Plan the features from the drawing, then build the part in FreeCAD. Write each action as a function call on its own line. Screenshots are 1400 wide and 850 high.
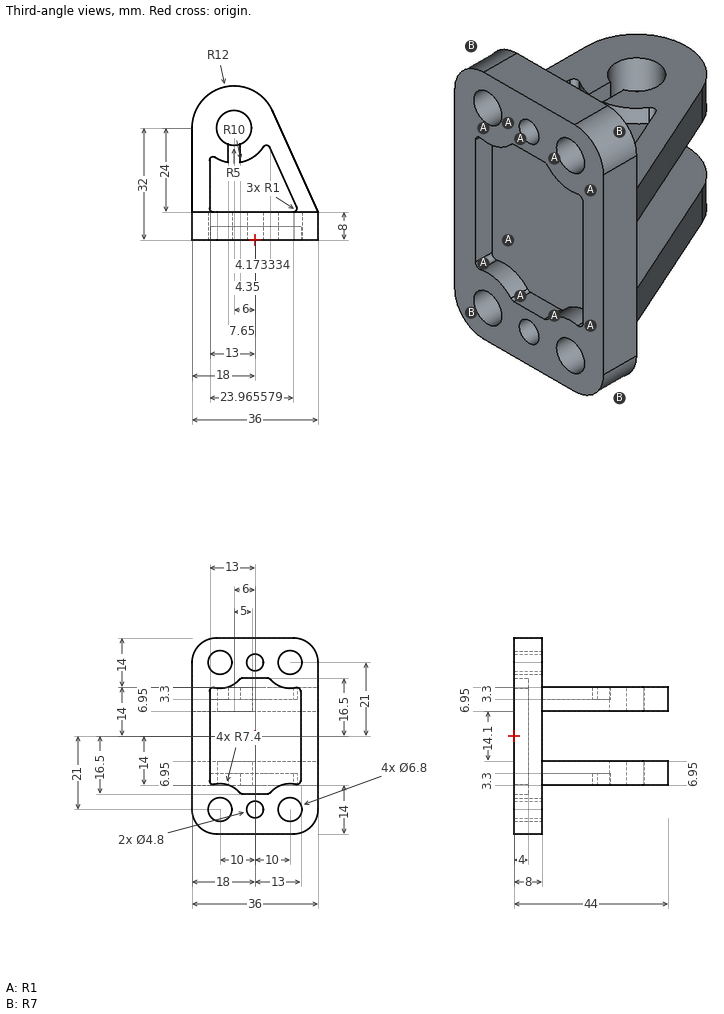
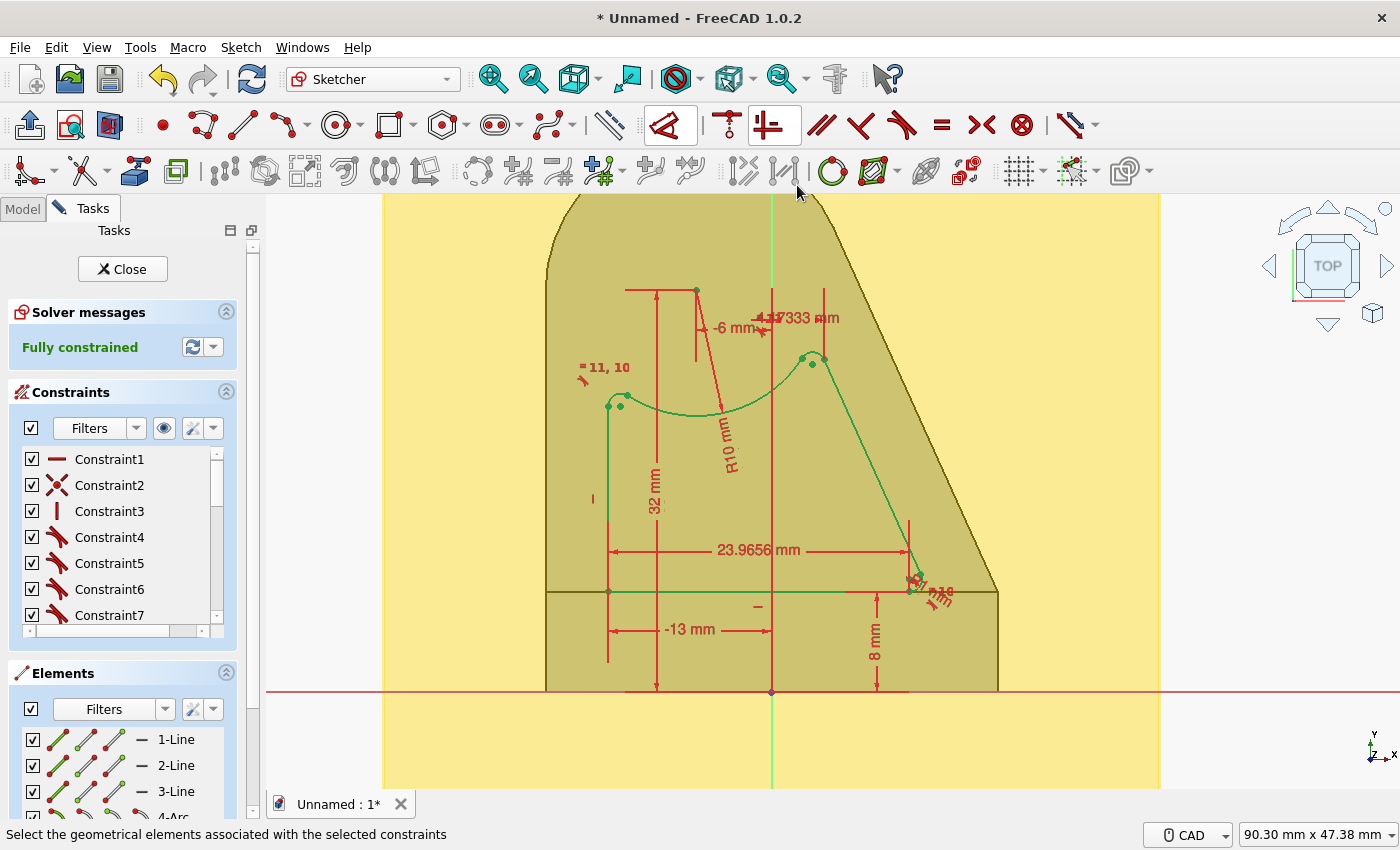
click(123, 269)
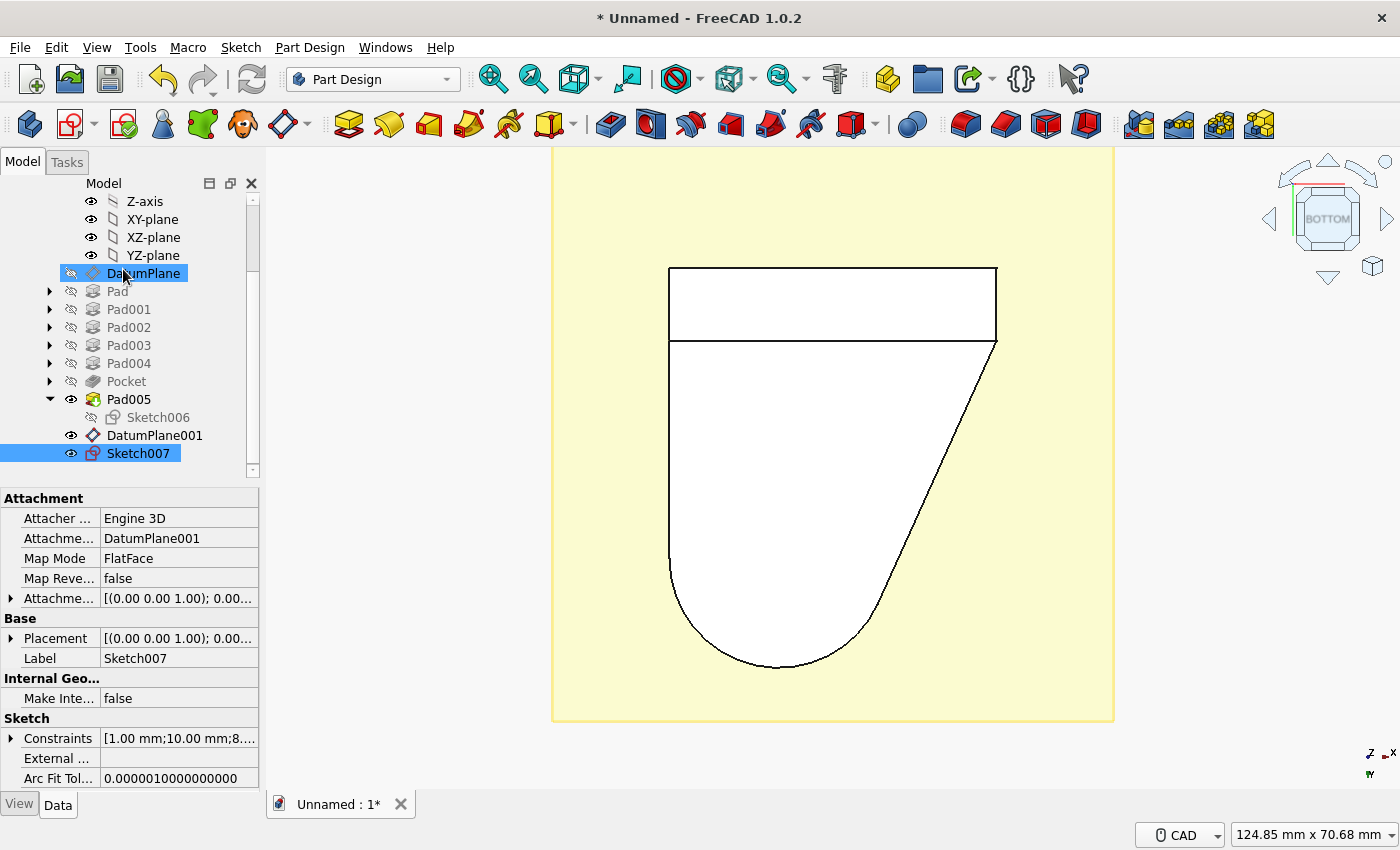
click(612, 124)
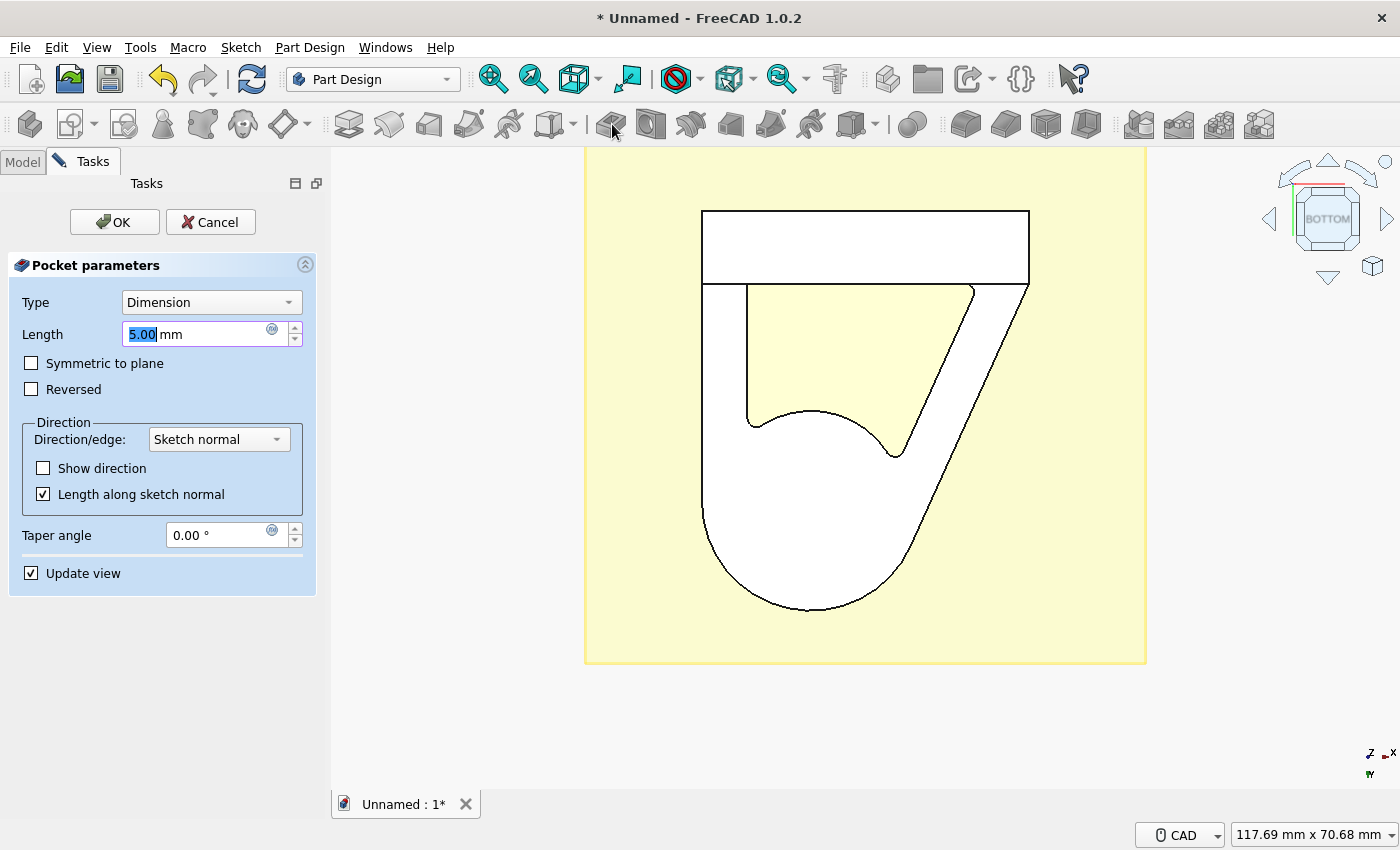
text(3.3)
key(Tab)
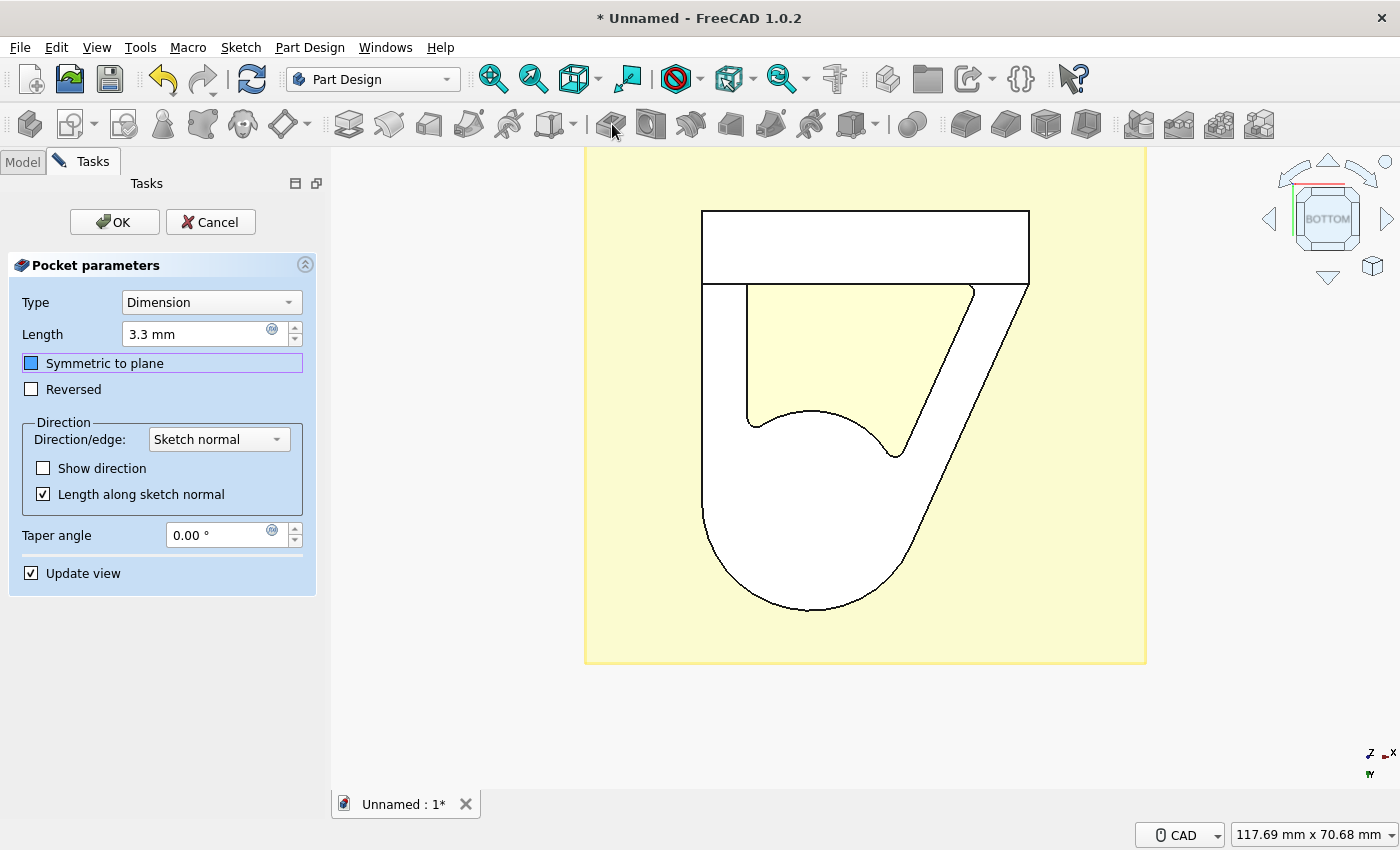
click(115, 222)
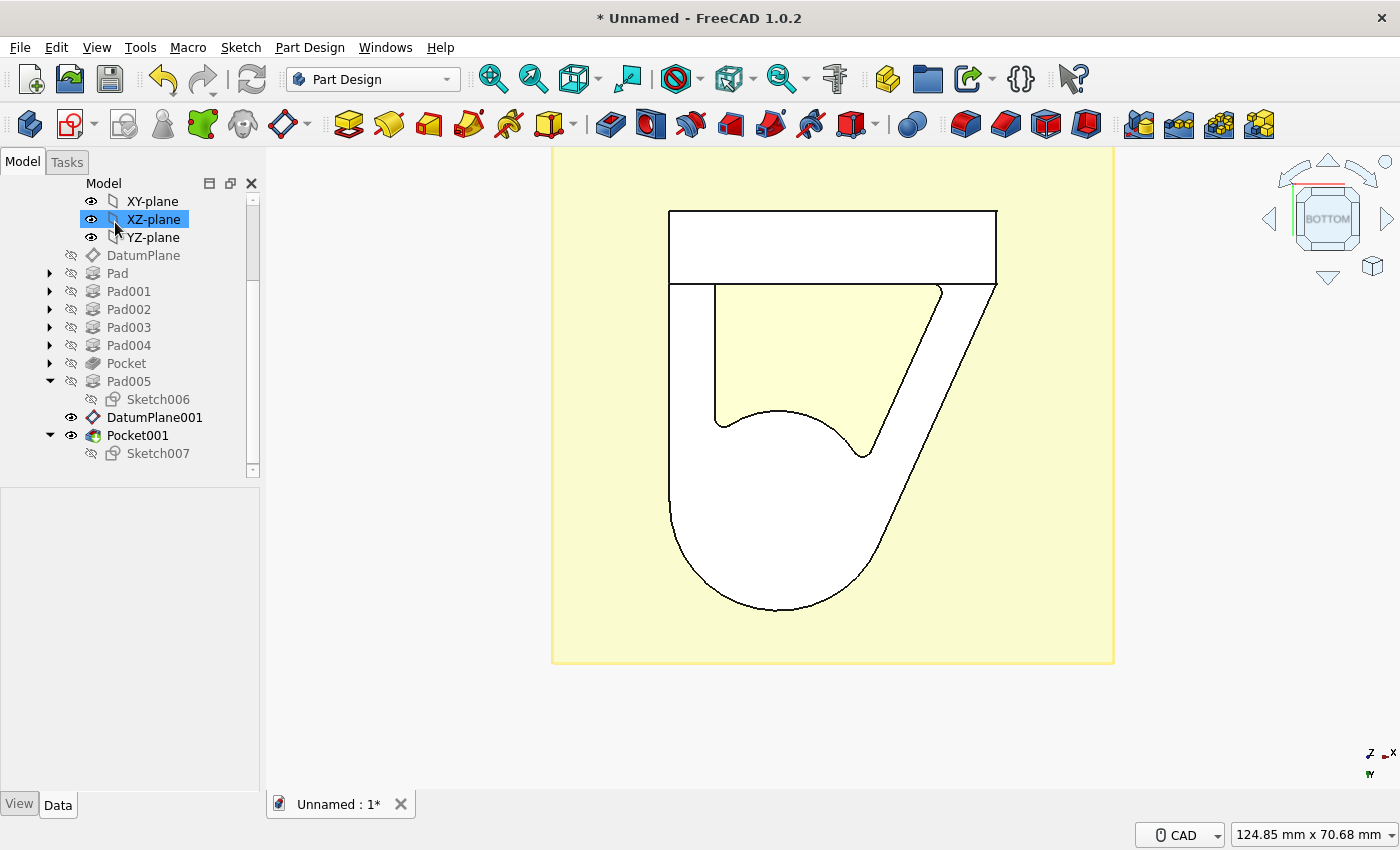
click(116, 417)
key(space)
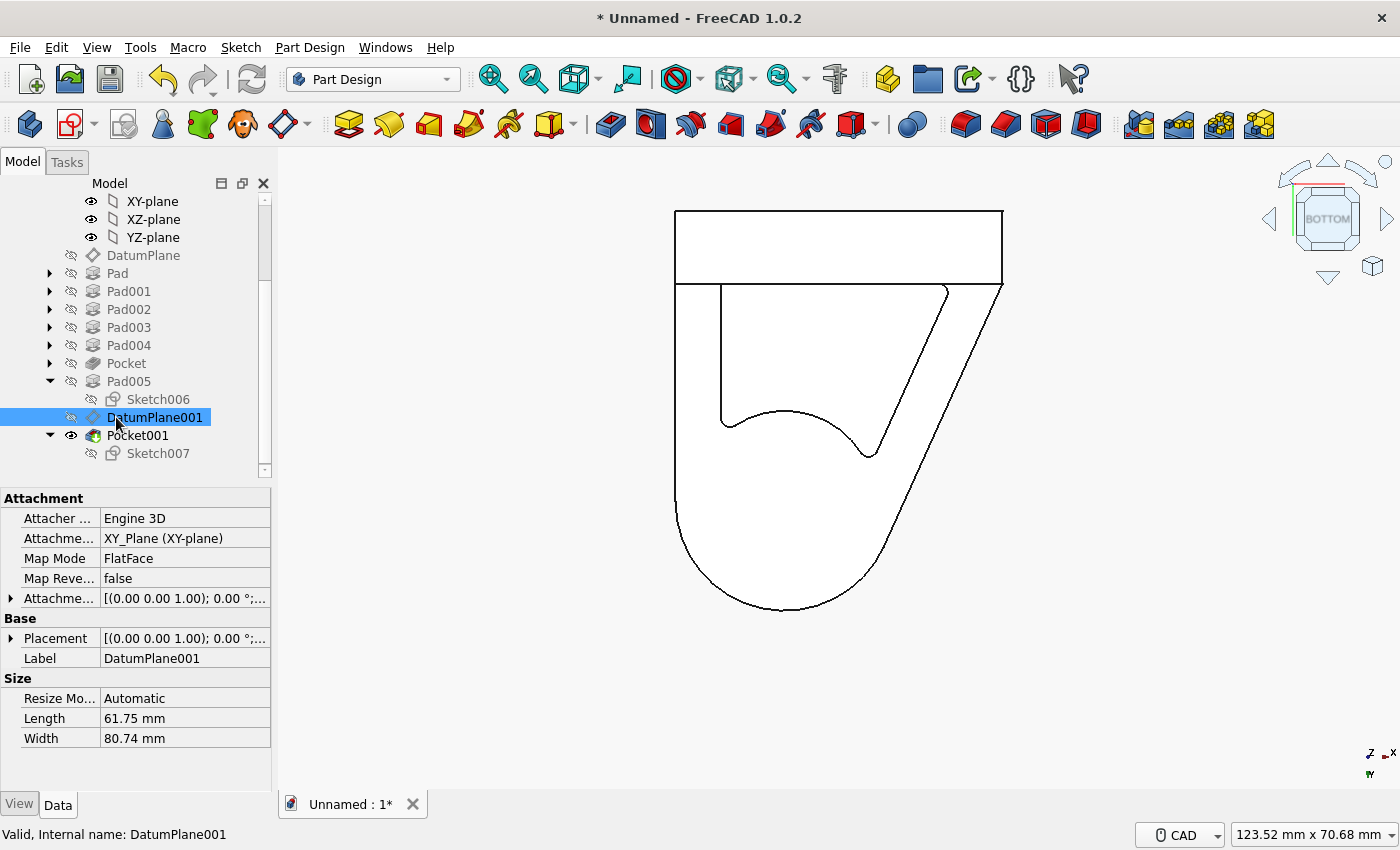
key(0)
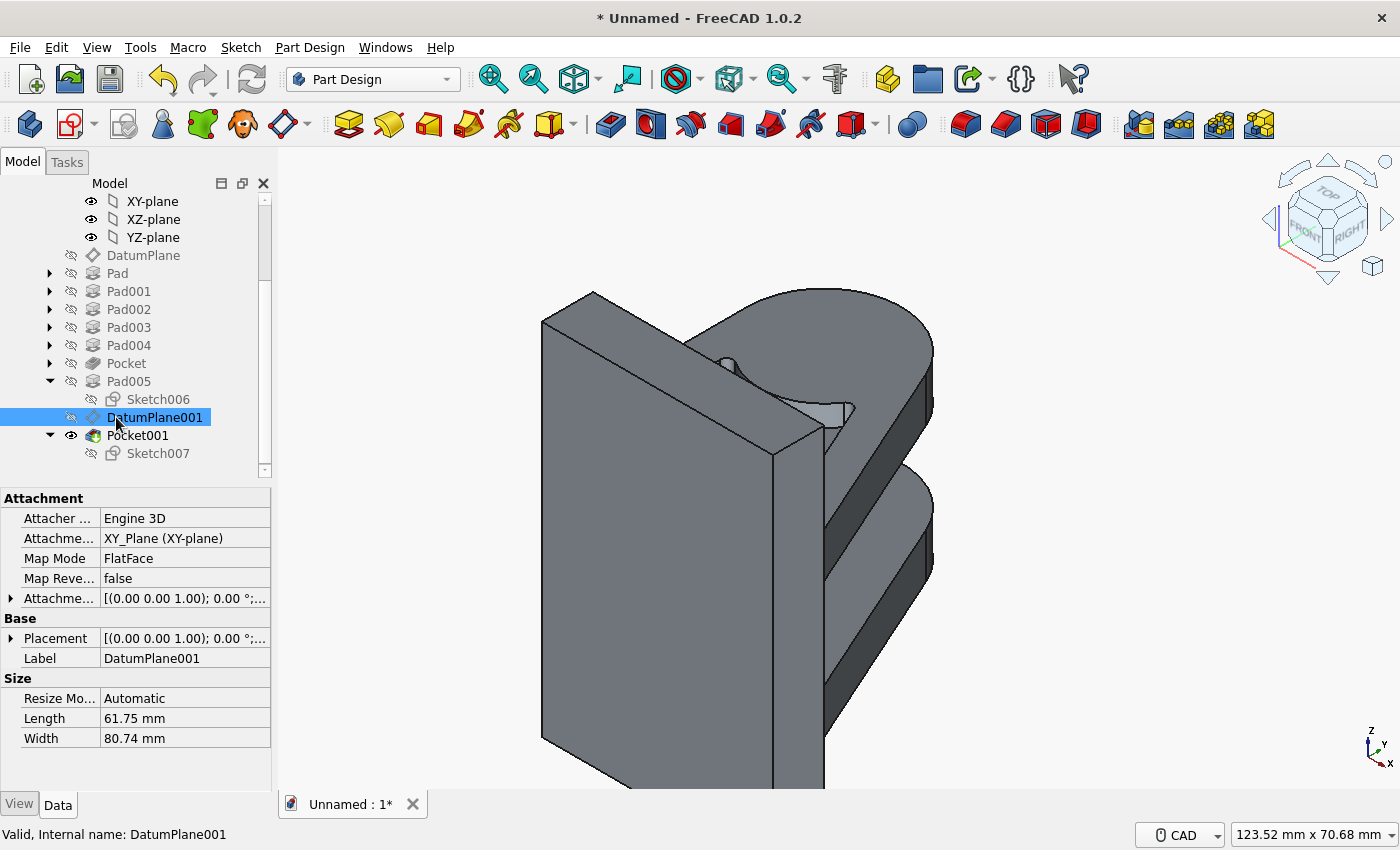
key(v)
key(f)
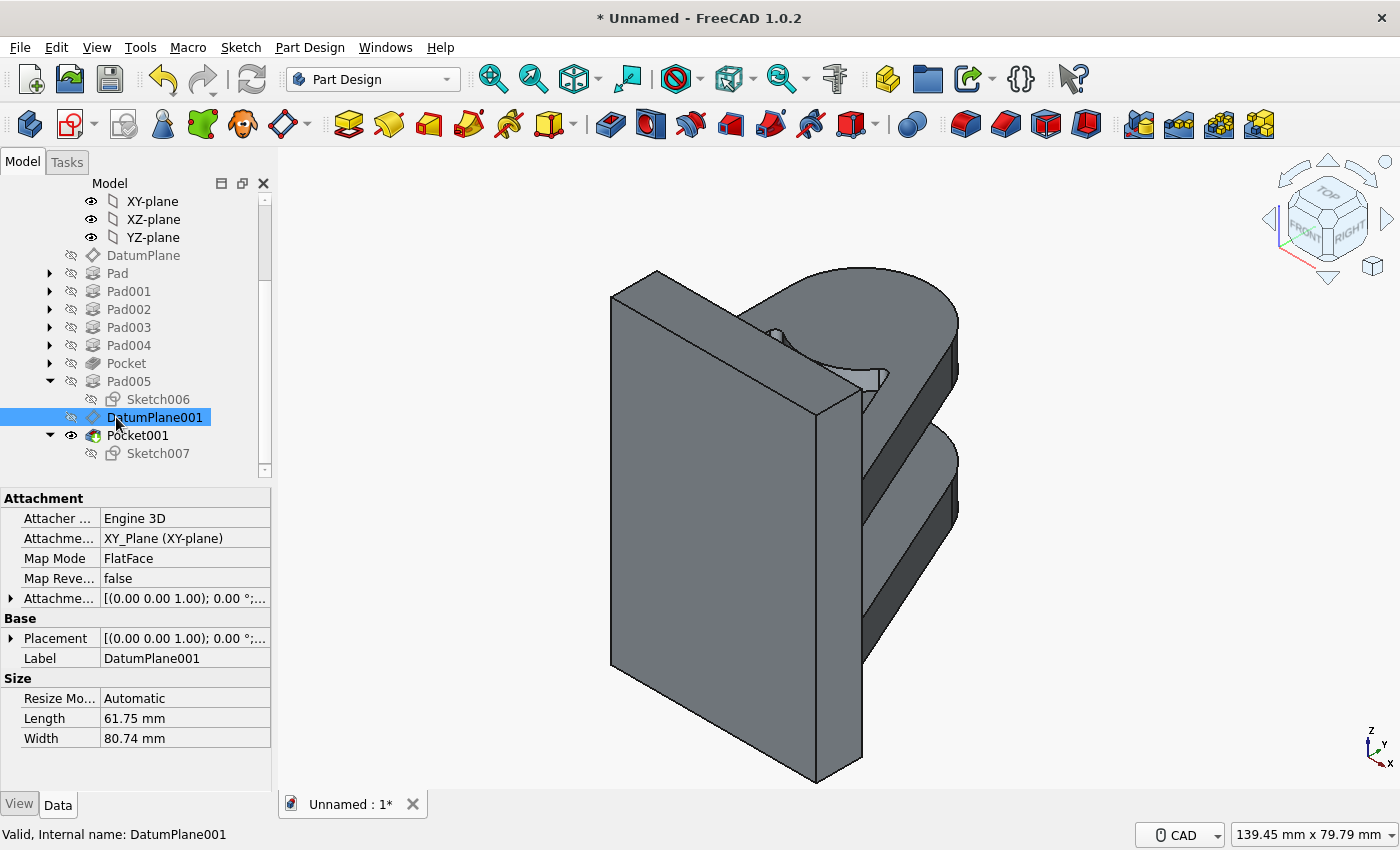
click(862, 328)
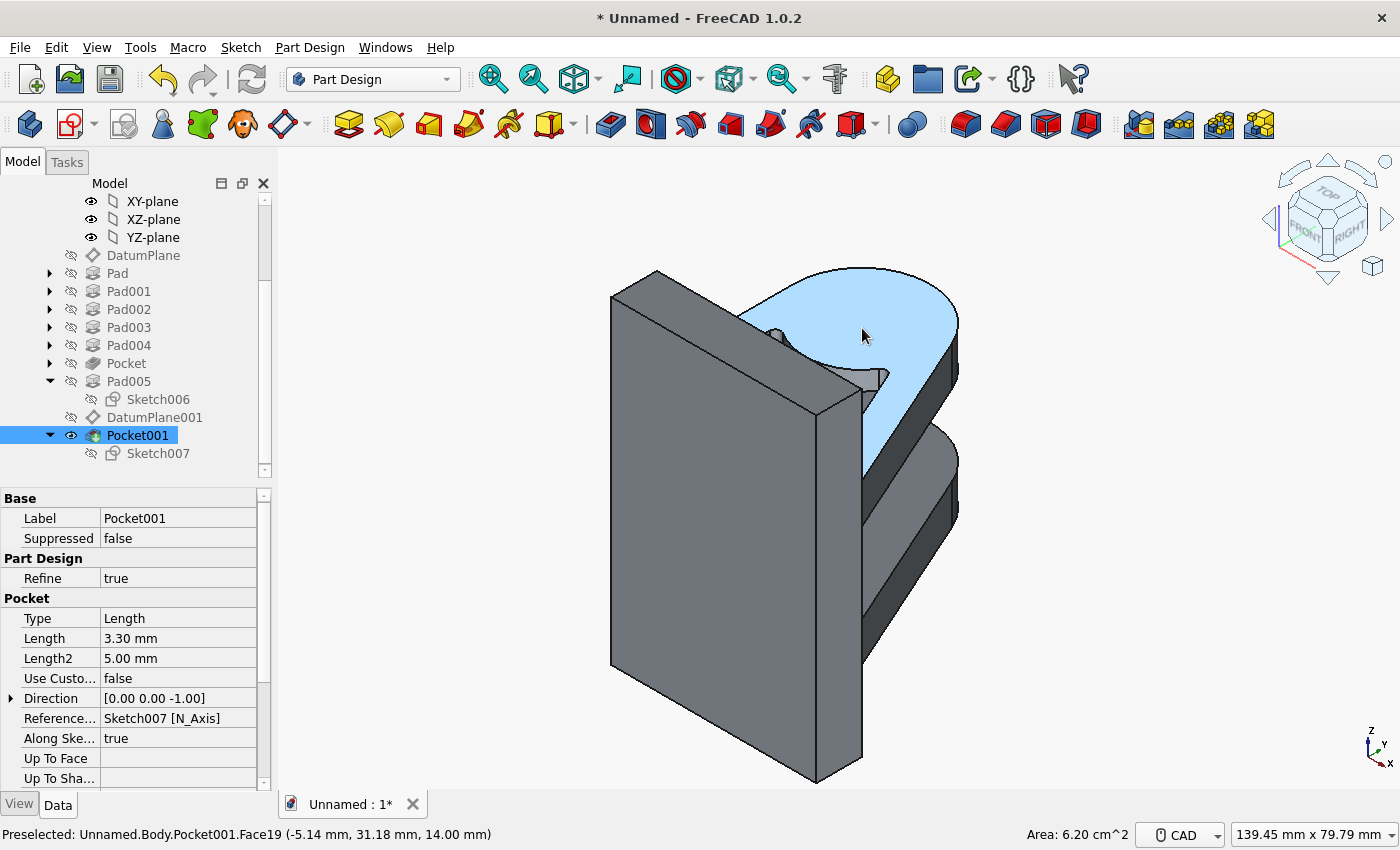
click(70, 124)